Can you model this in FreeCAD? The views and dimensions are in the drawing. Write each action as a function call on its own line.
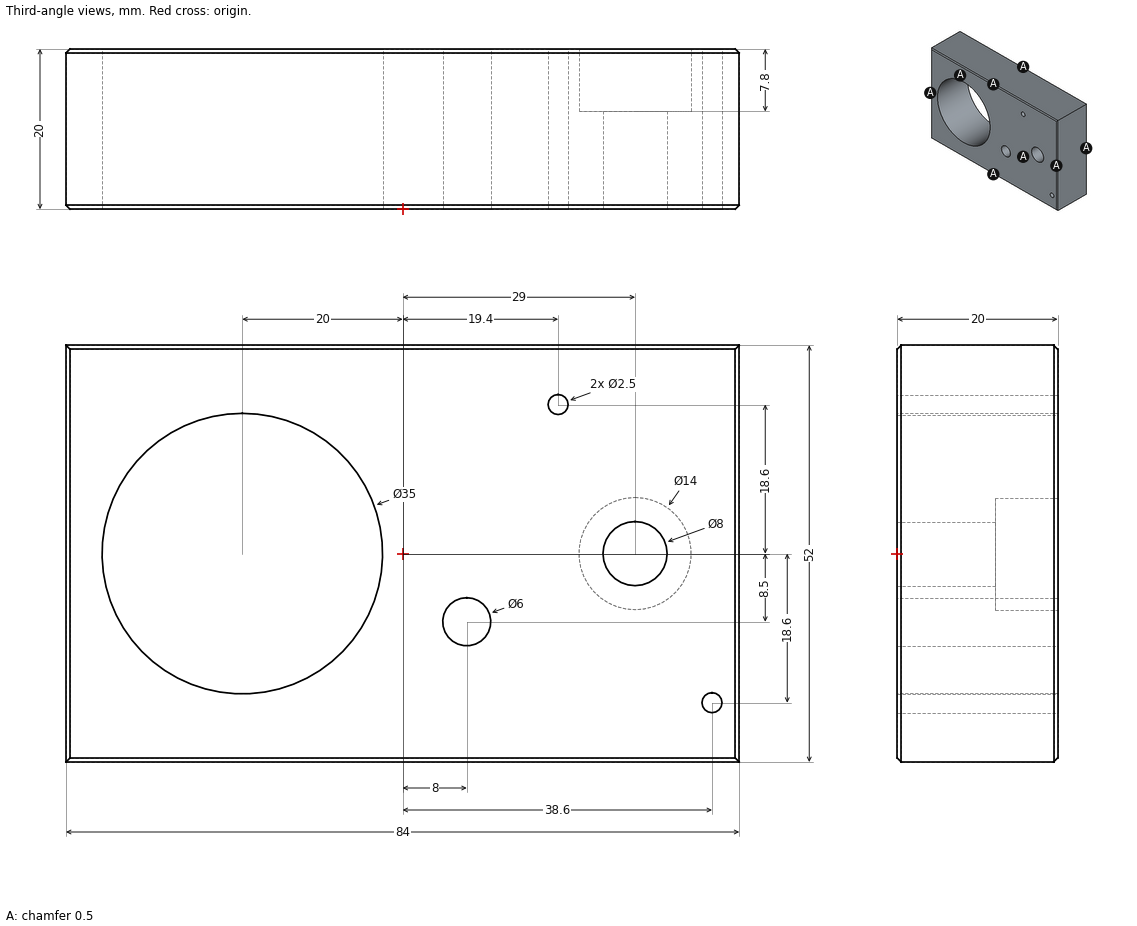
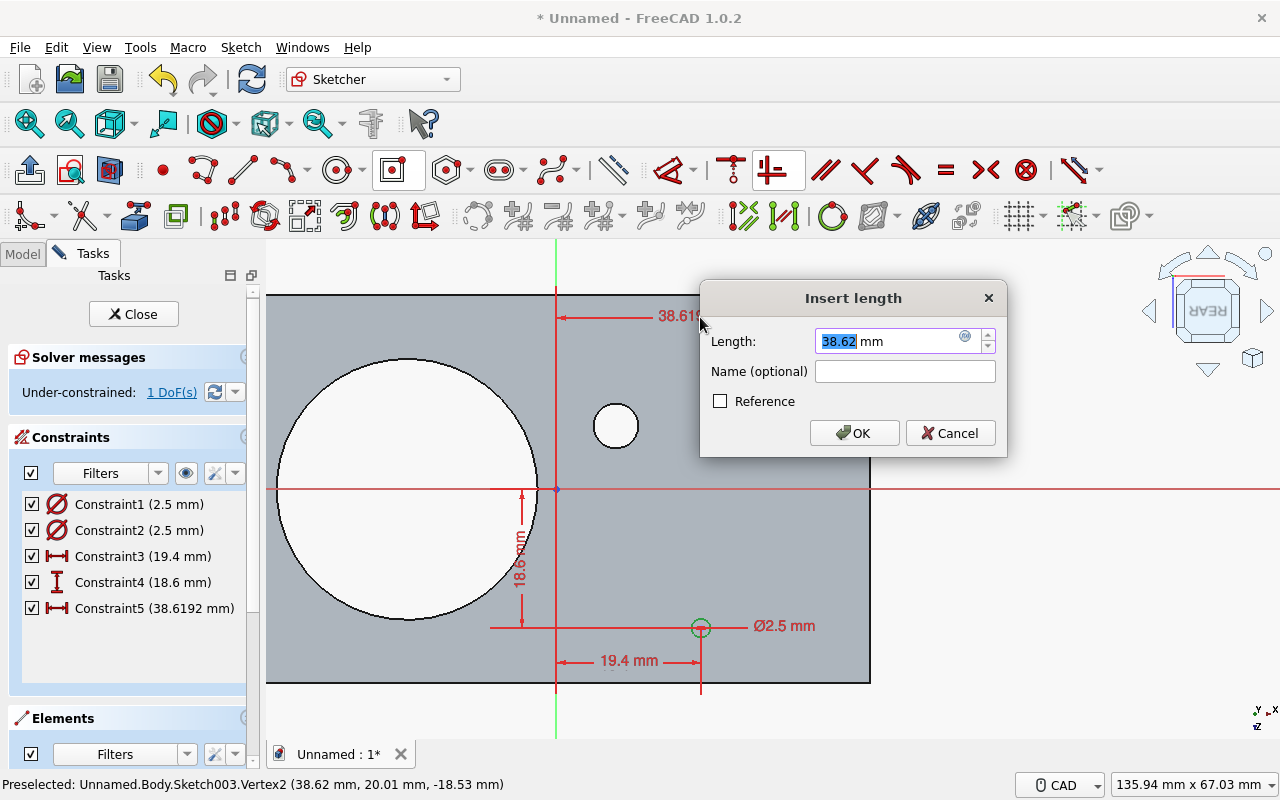
text(38.6)
key(Return)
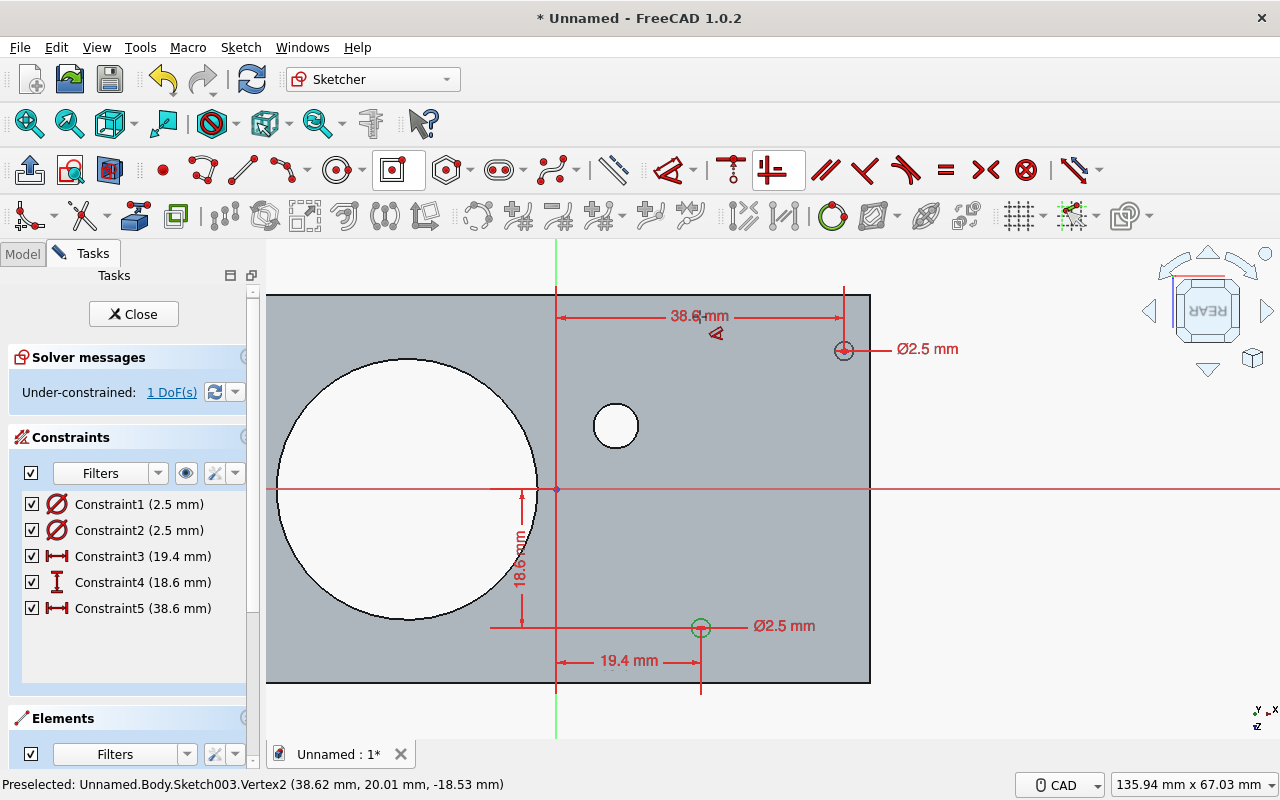
click(844, 351)
click(522, 420)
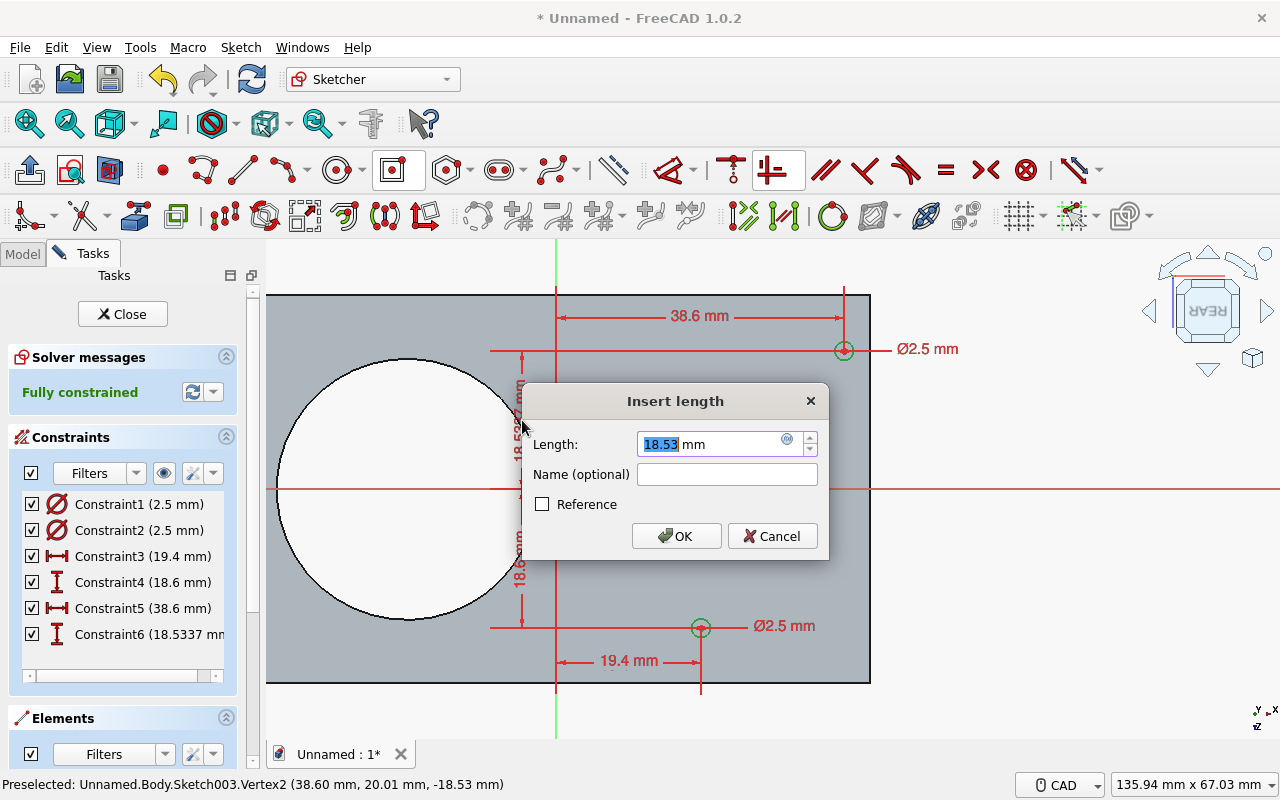
text(18.6)
key(Return)
key(Escape)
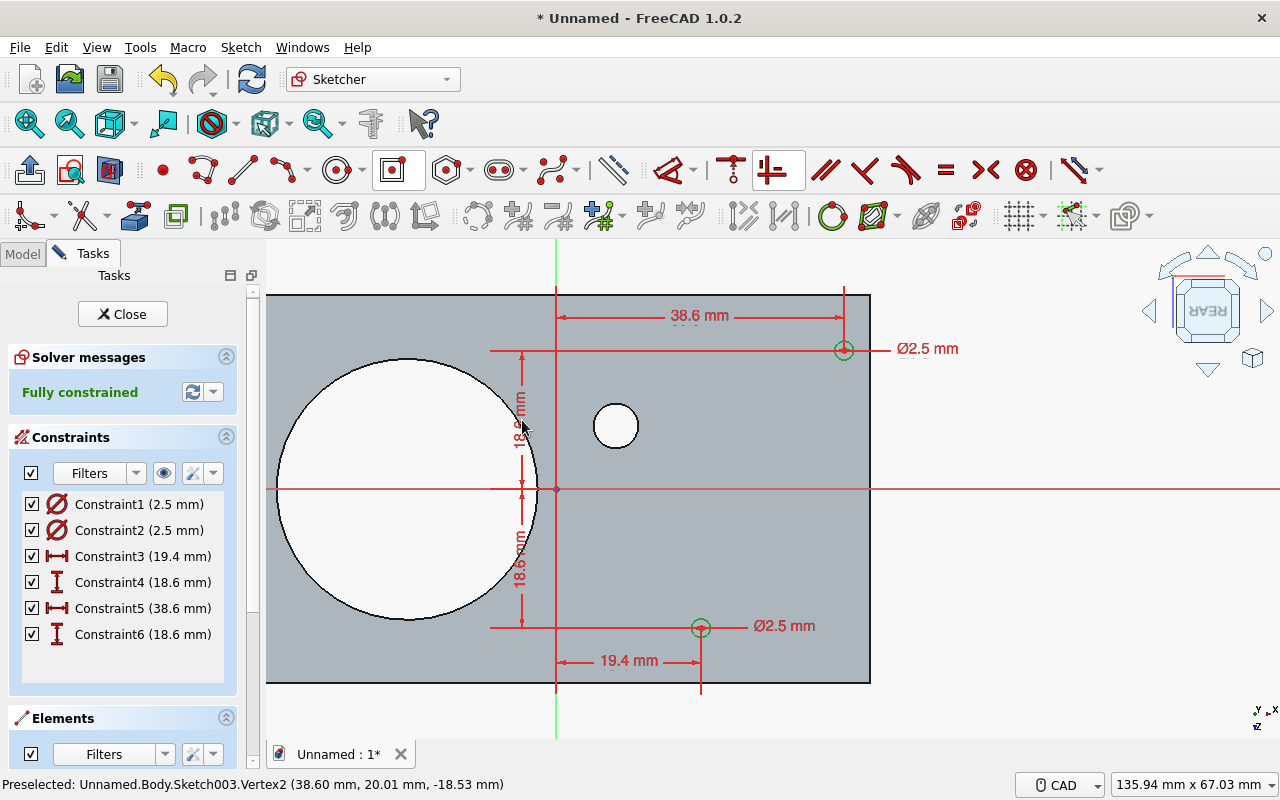
click(123, 314)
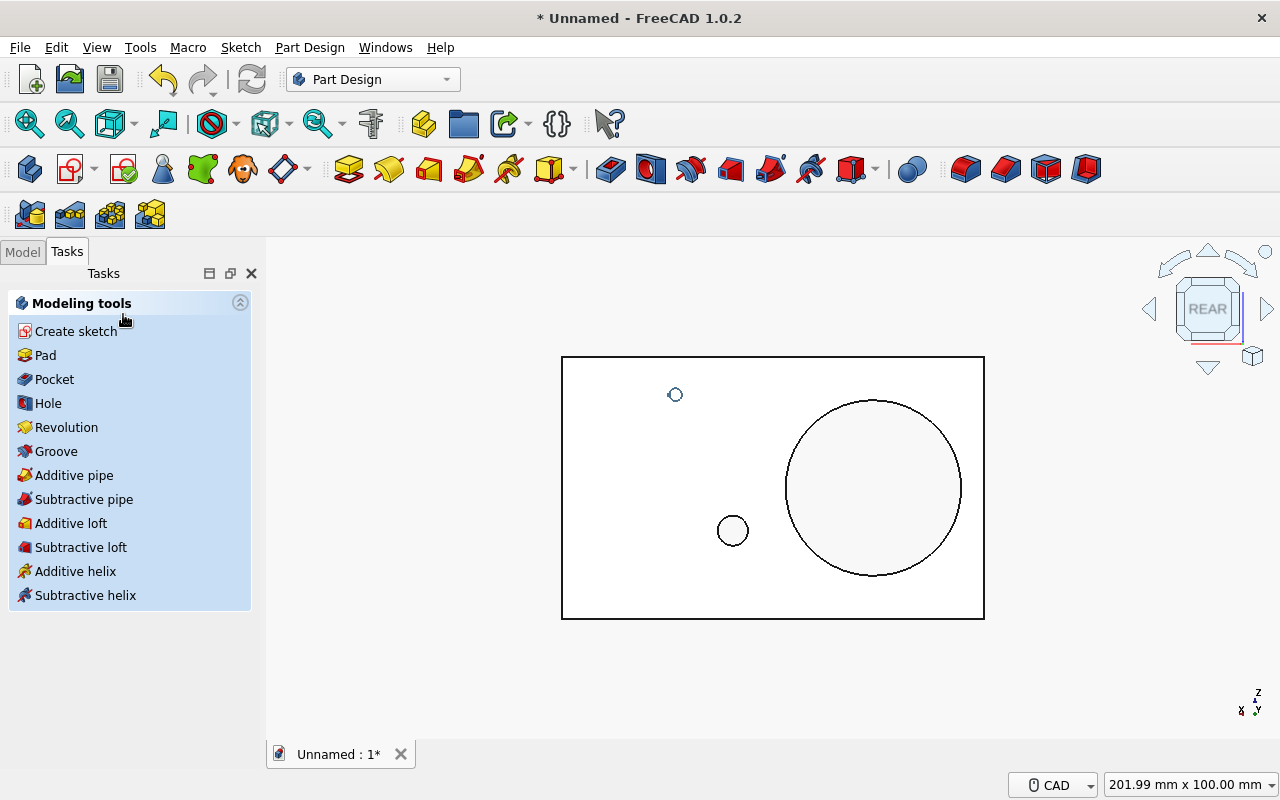
click(612, 170)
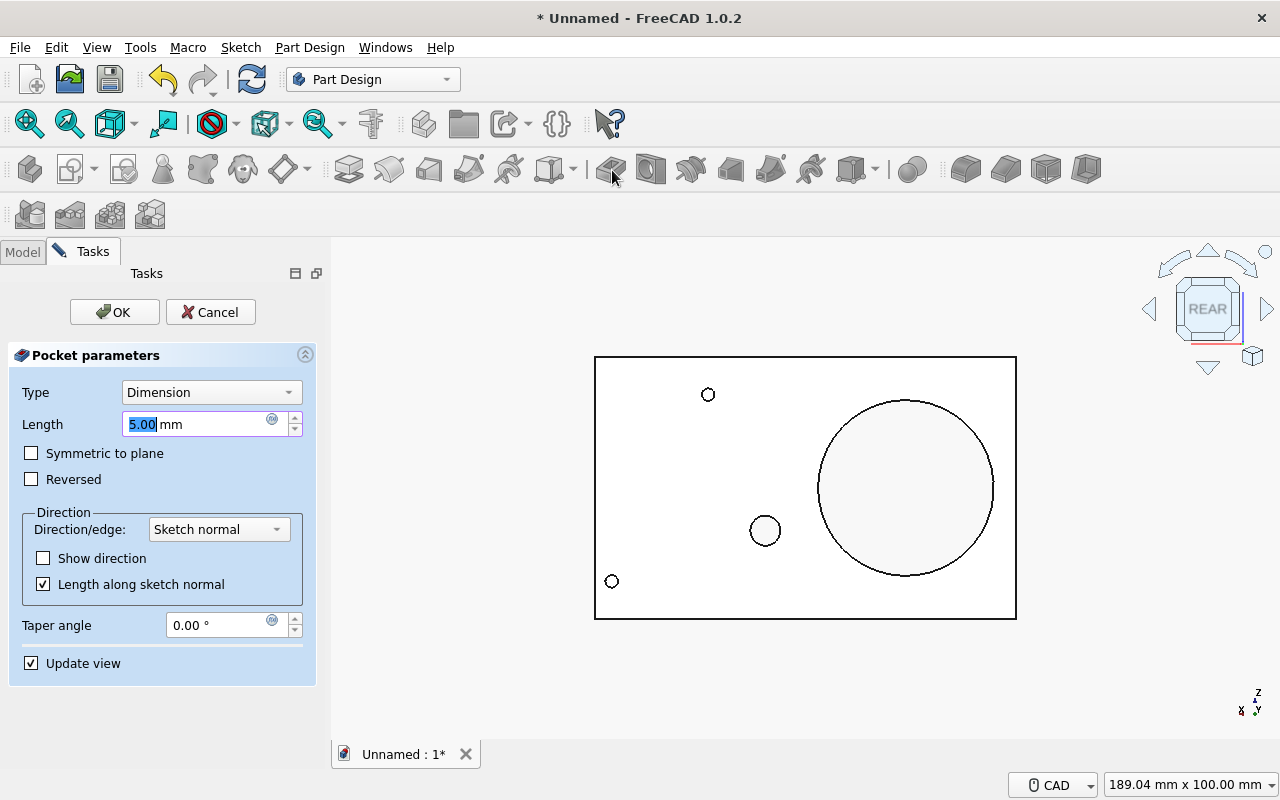
text(20)
key(Tab)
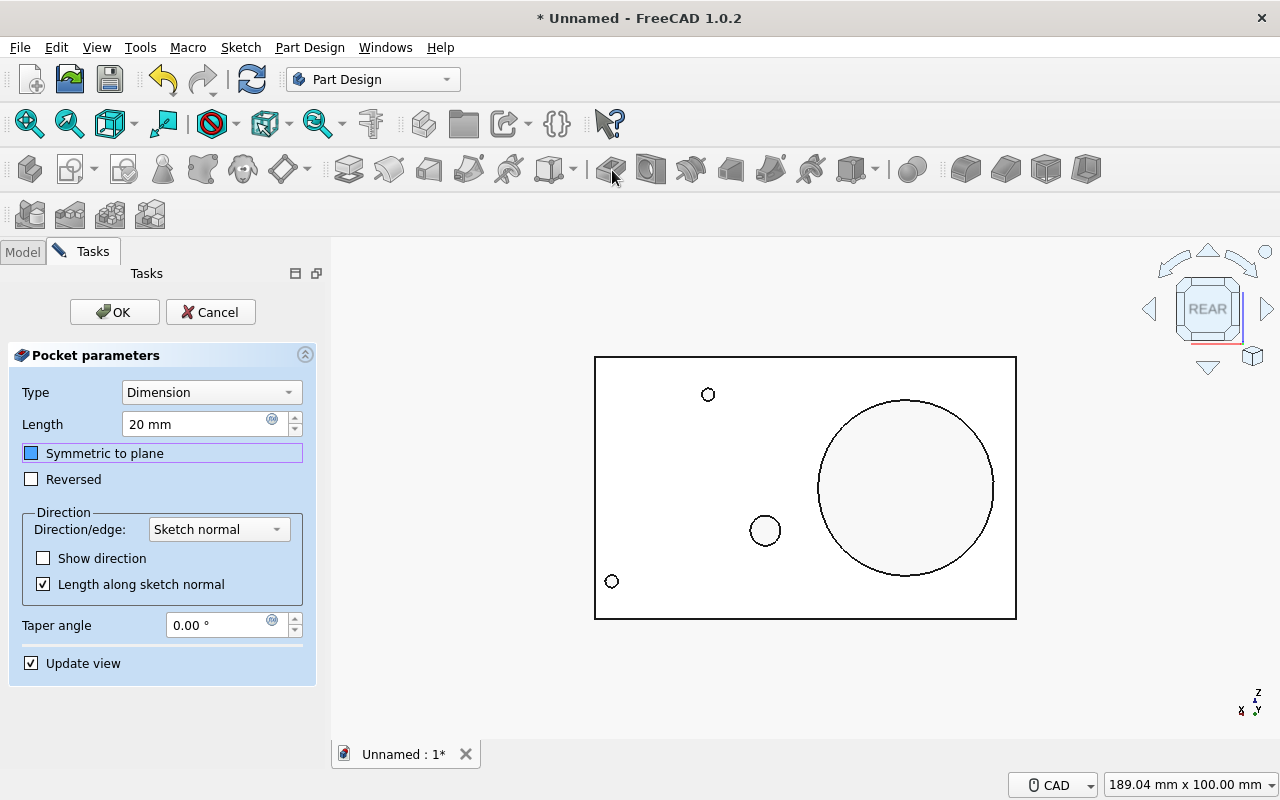
click(115, 312)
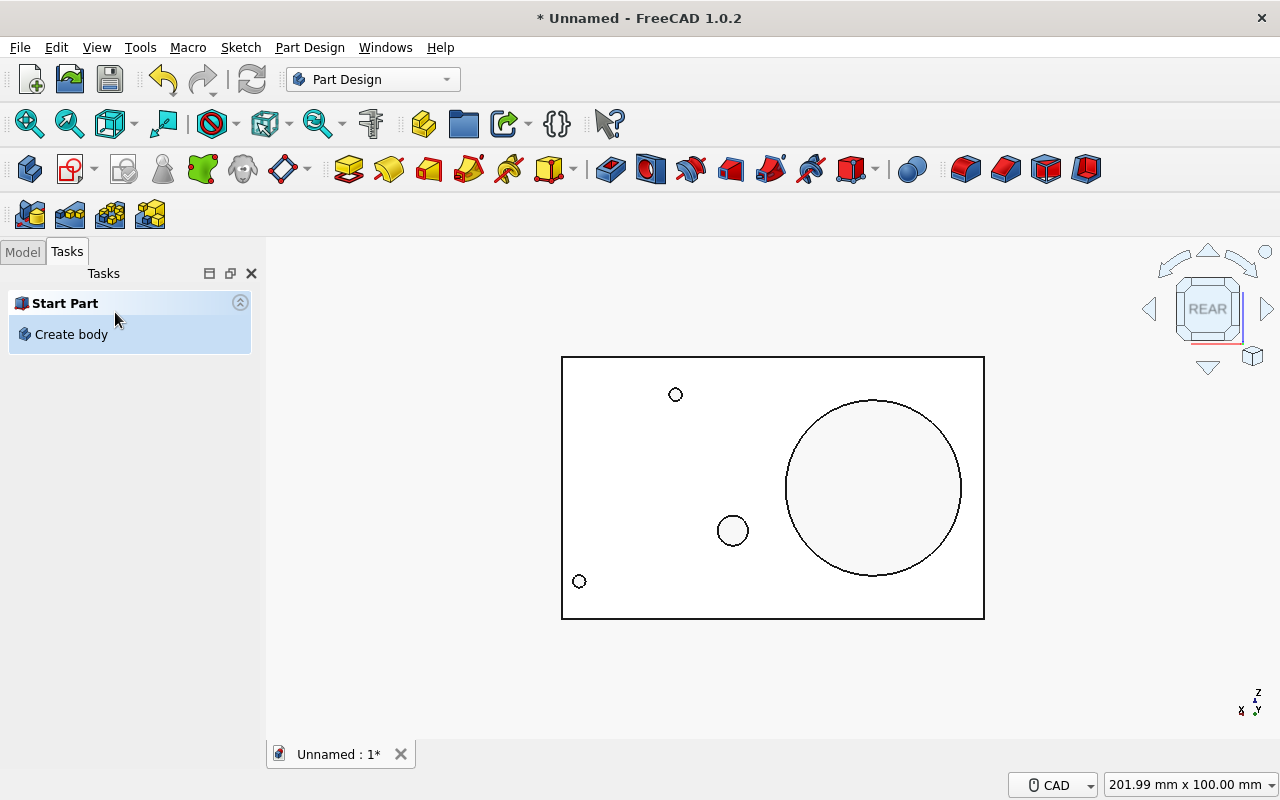
click(653, 487)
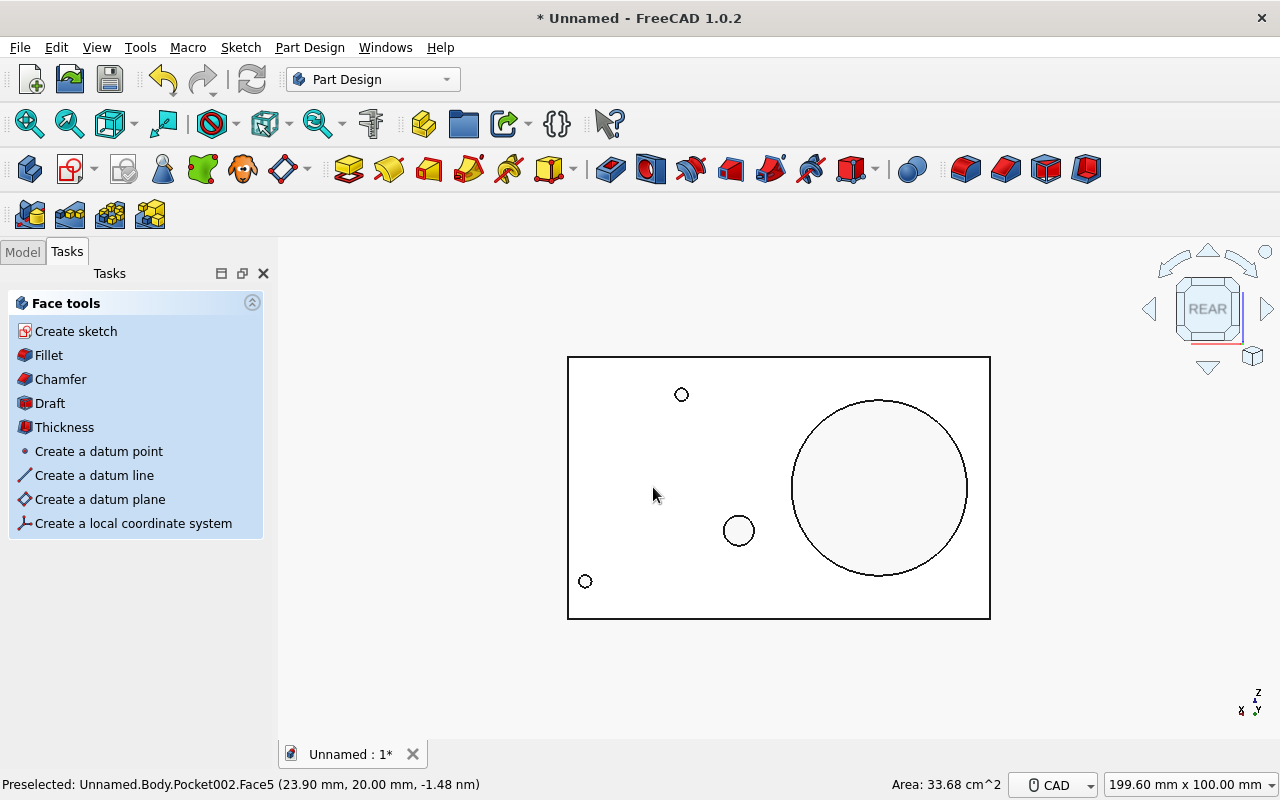
click(70, 170)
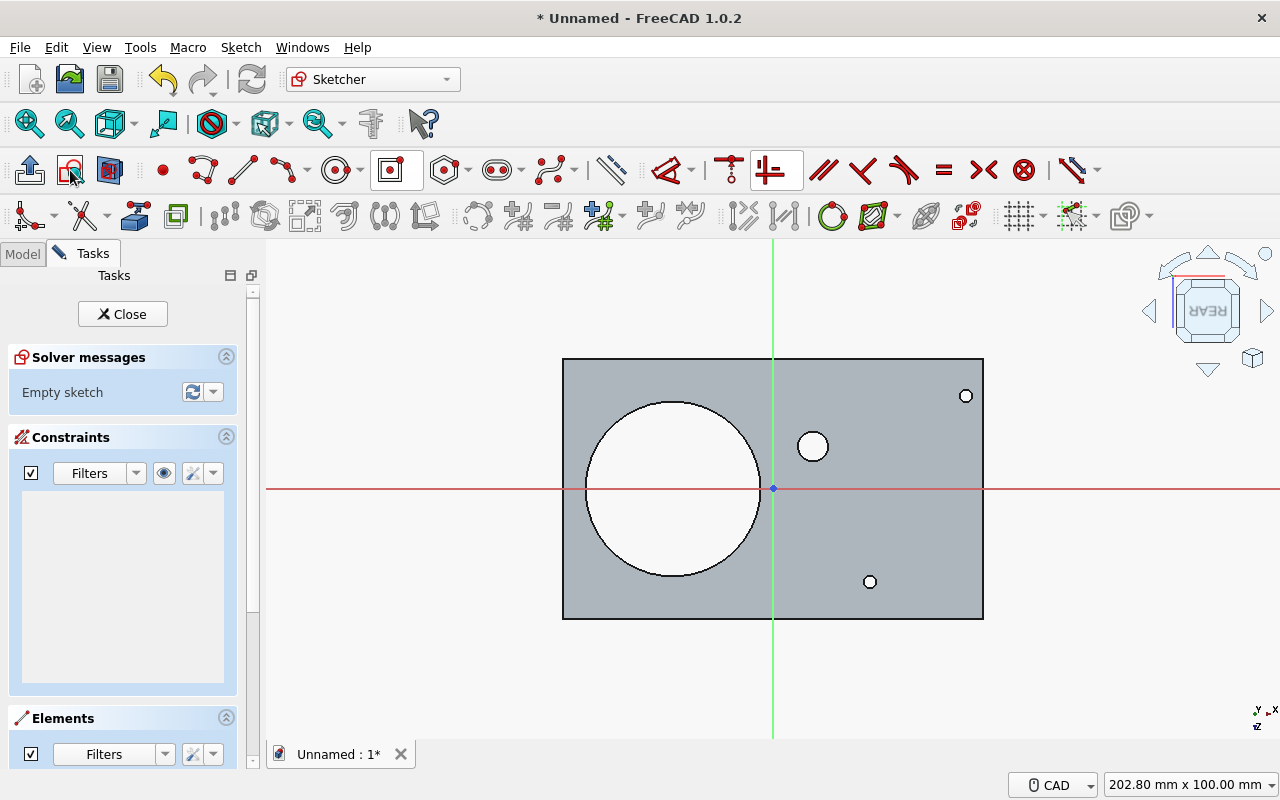
scroll(951, 489, up, 10)